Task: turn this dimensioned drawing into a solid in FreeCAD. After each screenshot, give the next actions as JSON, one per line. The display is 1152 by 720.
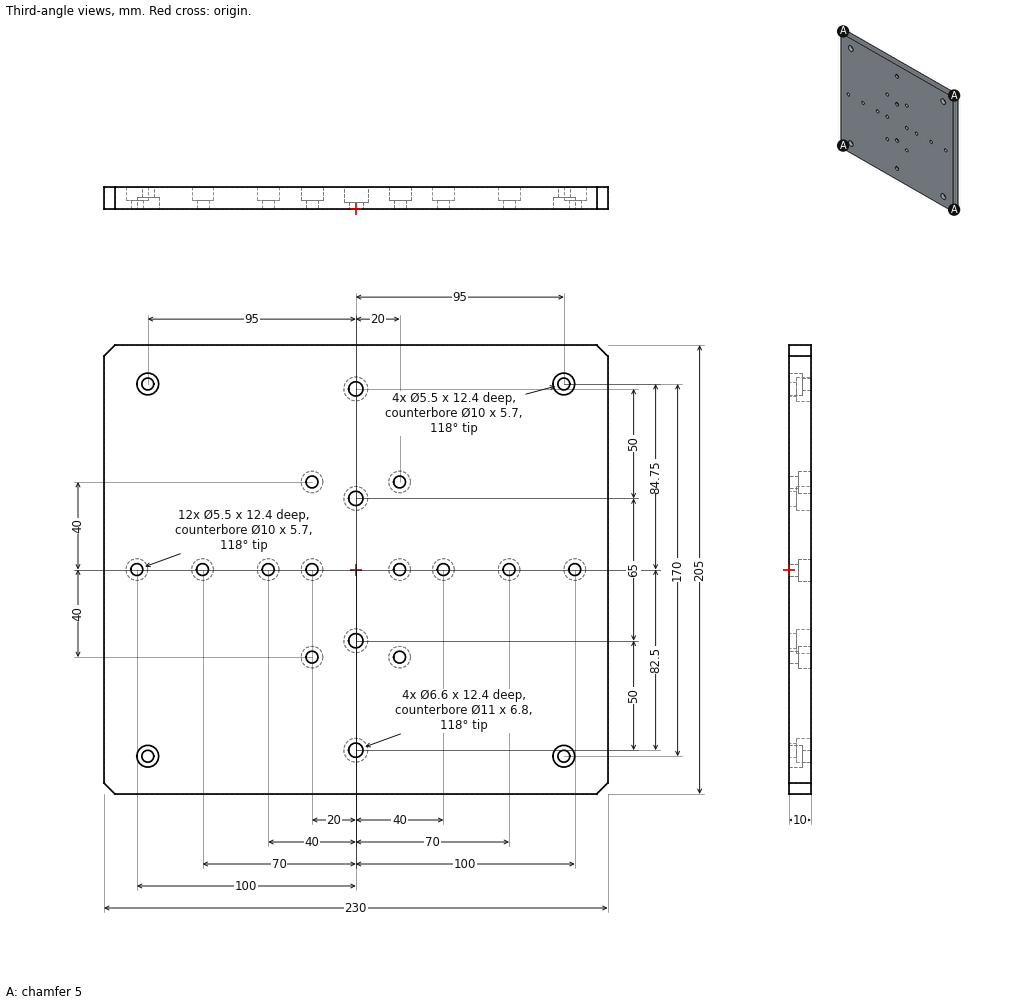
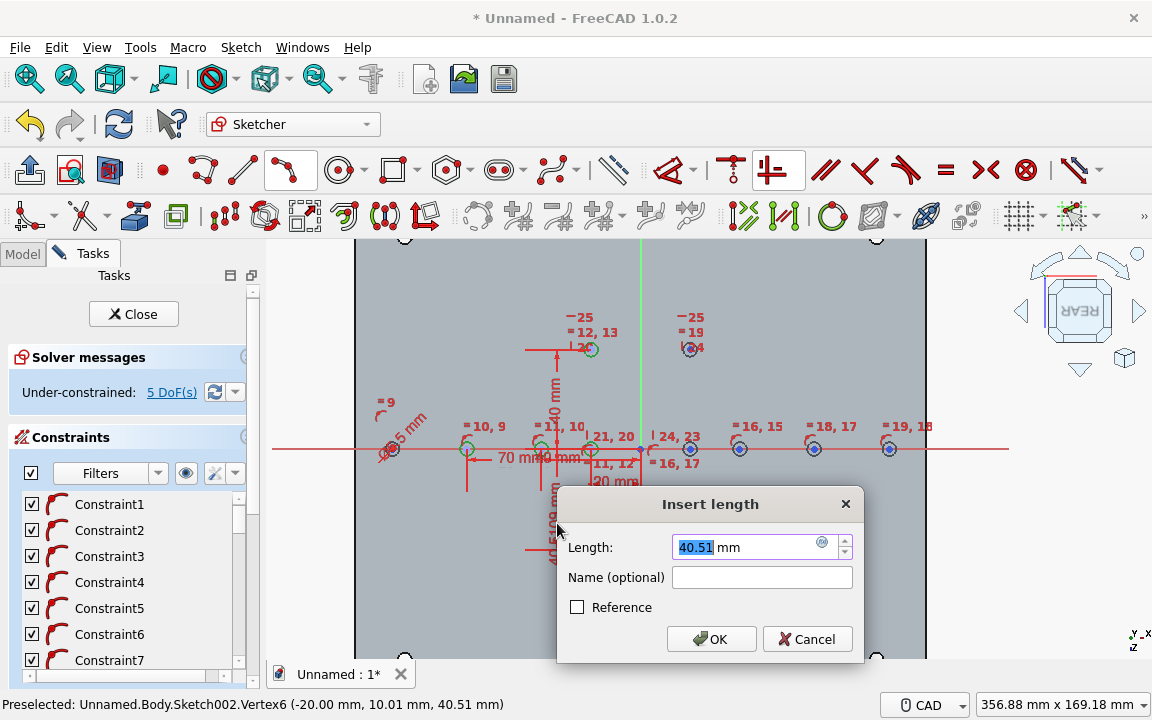
{"action": "type", "text": "40"}
{"action": "key", "text": "Return"}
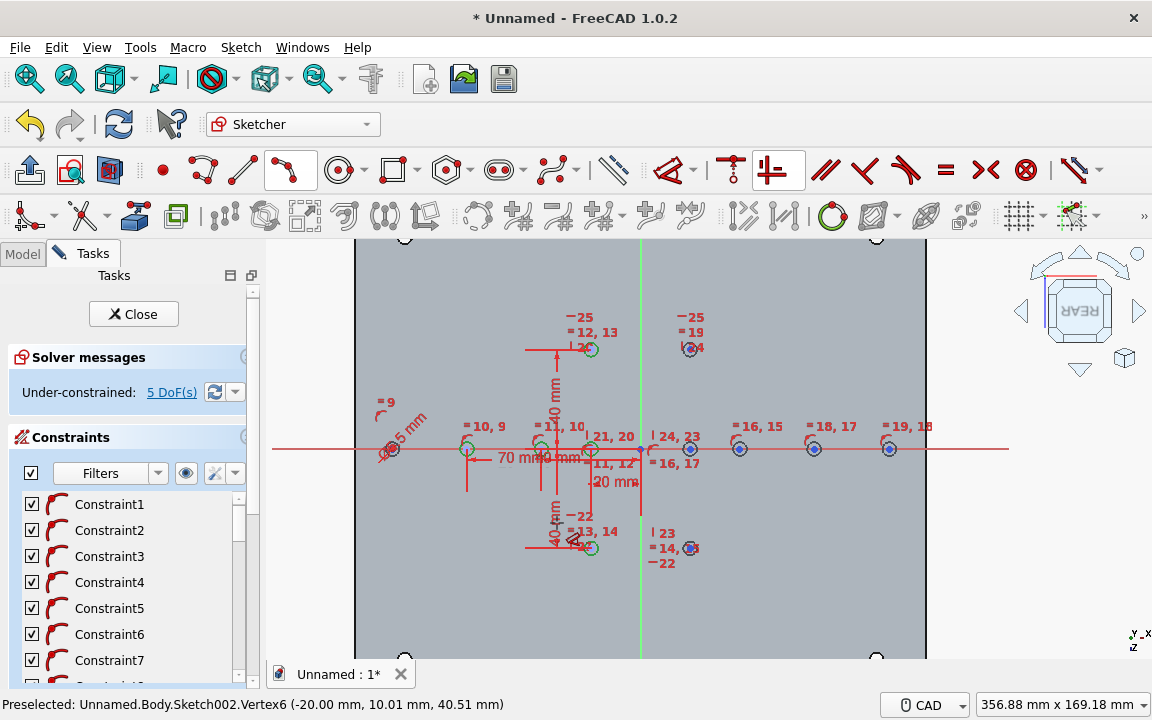
{"action": "left_click", "coordinate": [690, 548]}
{"action": "left_click", "coordinate": [665, 582]}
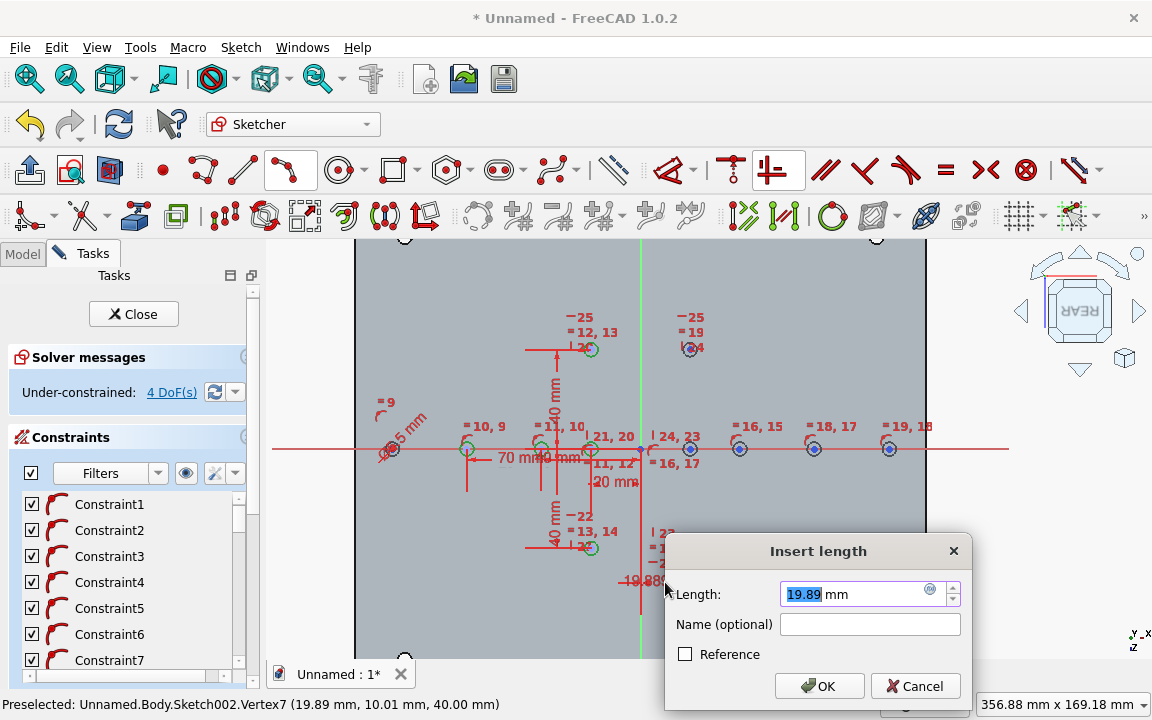
{"action": "type", "text": "20"}
{"action": "key", "text": "Return"}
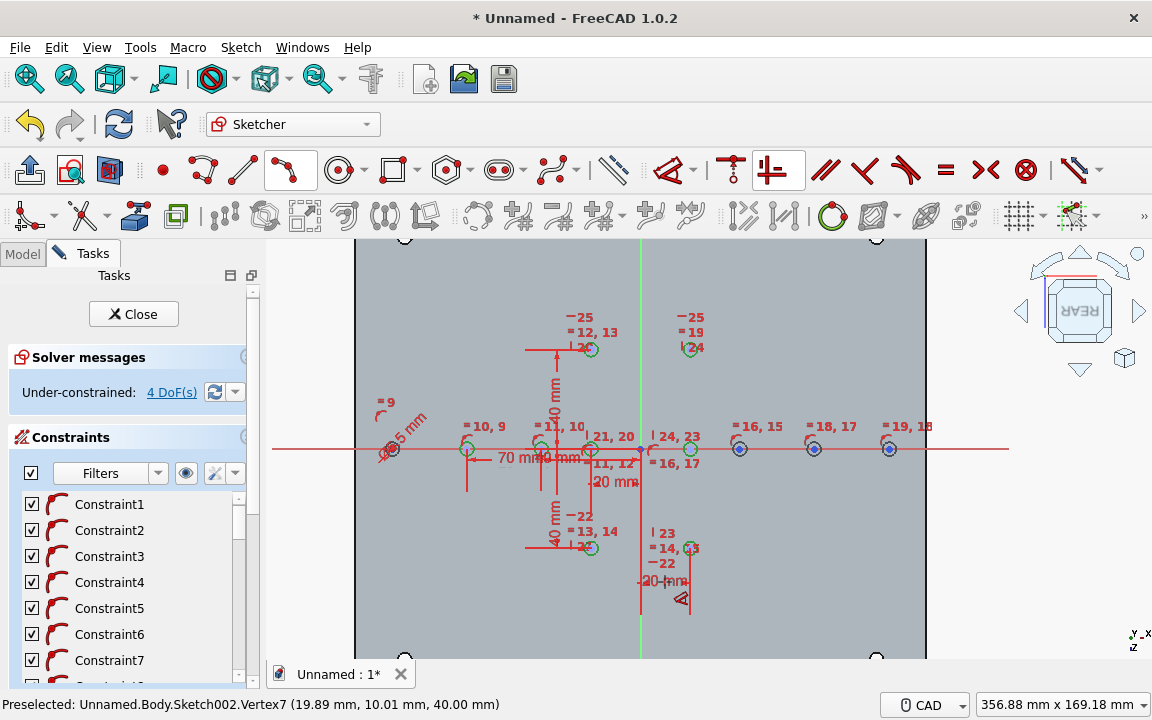
{"action": "left_click", "coordinate": [740, 449]}
{"action": "left_click", "coordinate": [690, 483]}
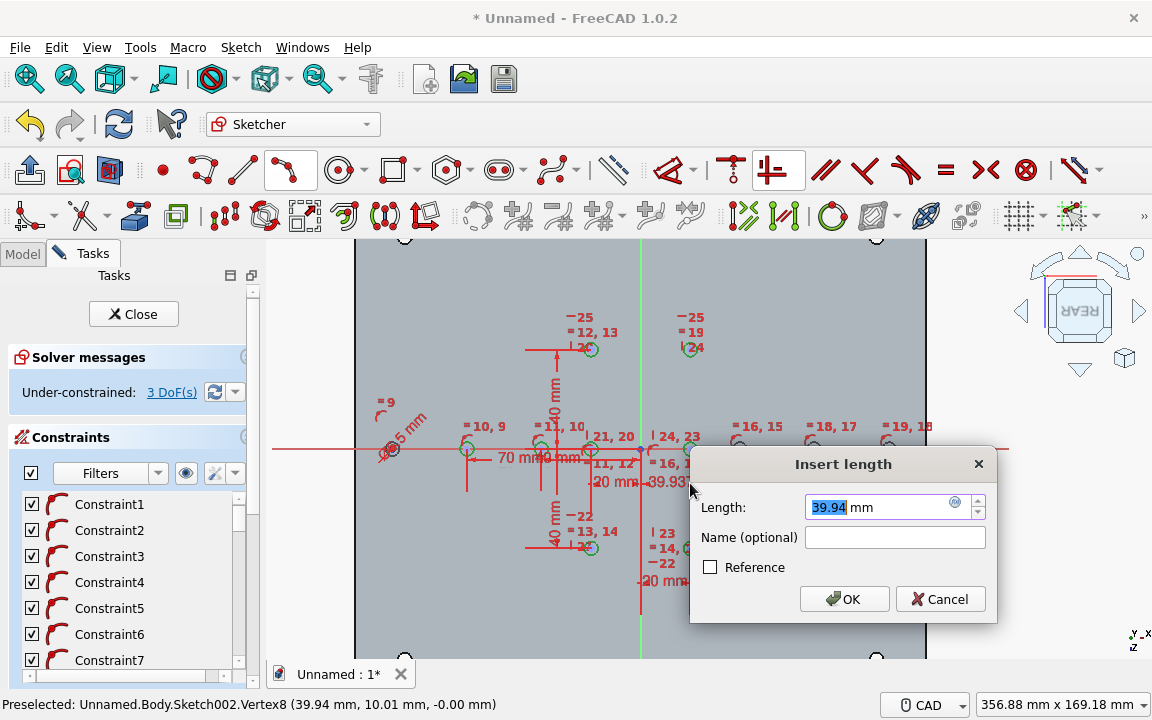
{"action": "type", "text": "40"}
{"action": "key", "text": "Return"}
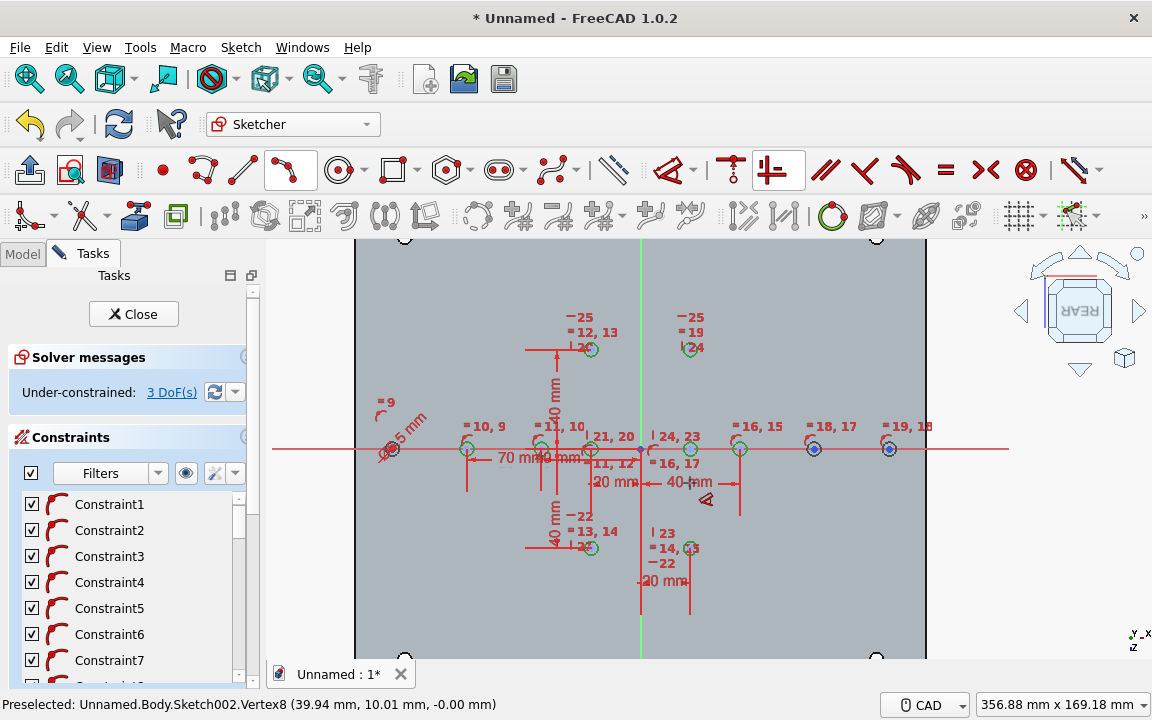
{"action": "left_click", "coordinate": [814, 449]}
{"action": "left_click", "coordinate": [767, 483]}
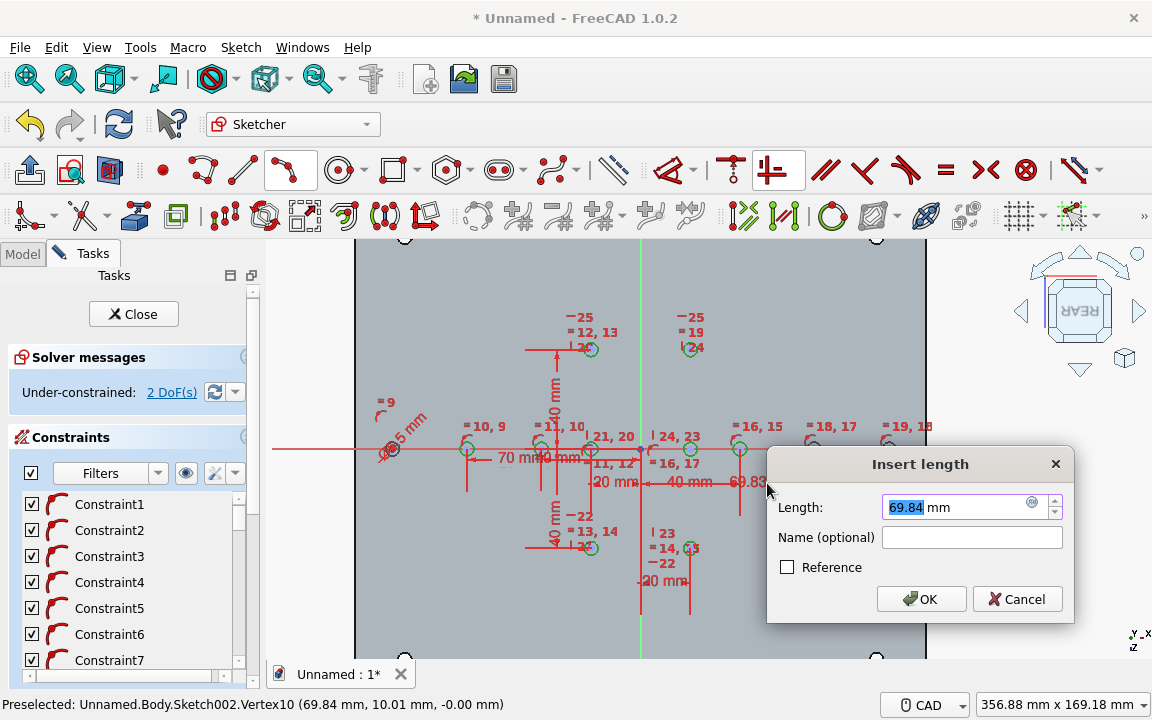
{"action": "type", "text": "70"}
{"action": "key", "text": "Return"}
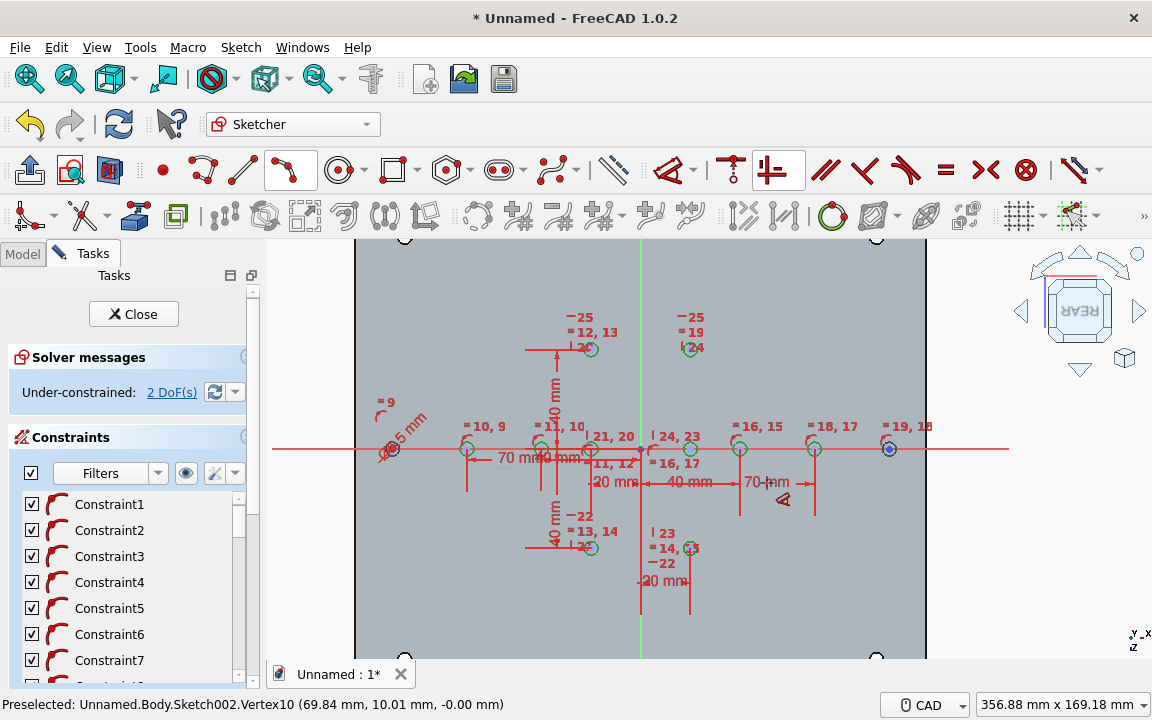
{"action": "left_click", "coordinate": [393, 449]}
{"action": "left_click", "coordinate": [517, 483]}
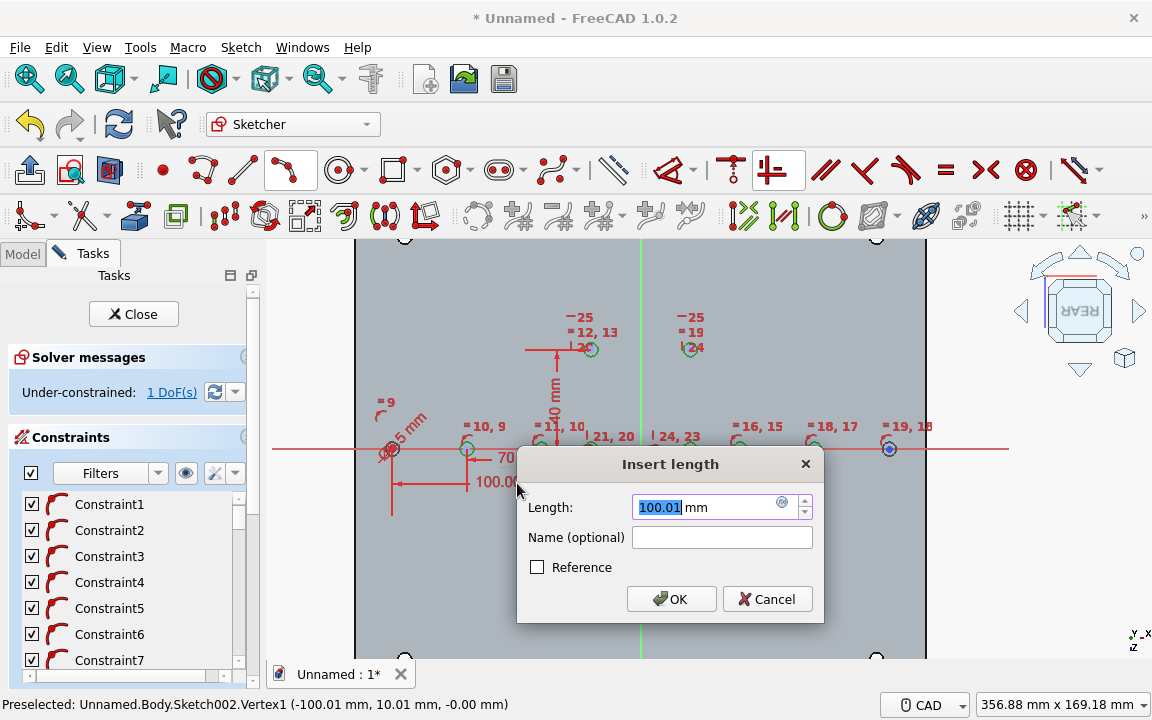
{"action": "type", "text": "100"}
{"action": "key", "text": "Return"}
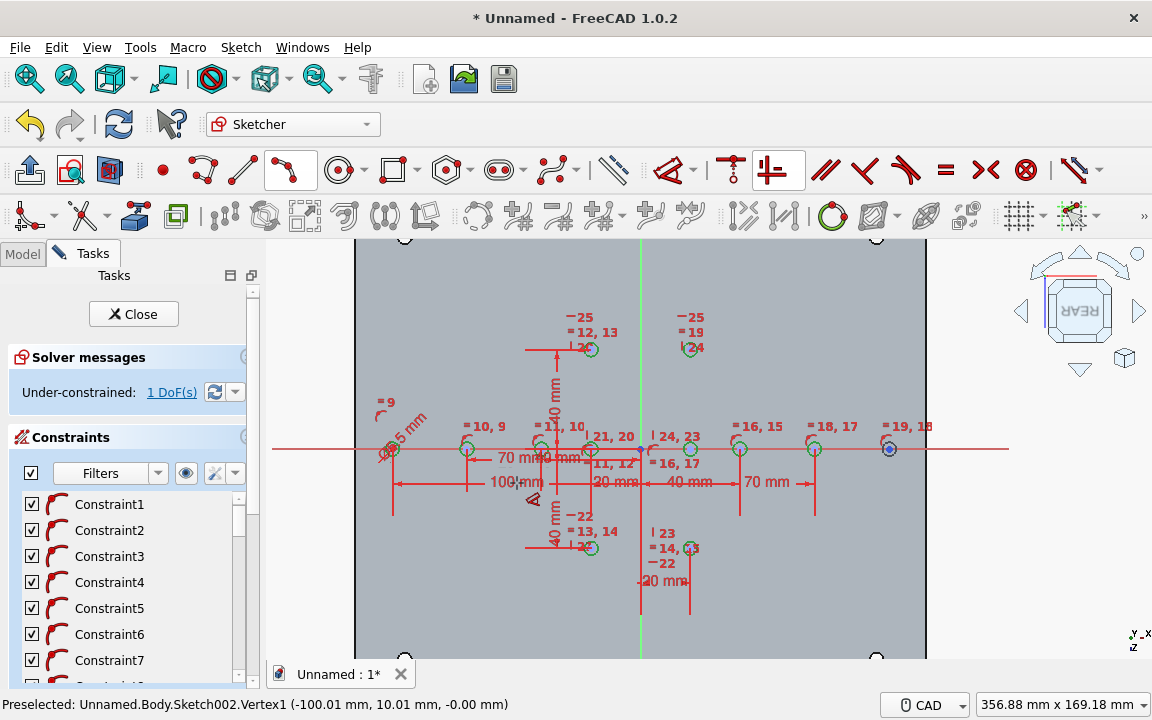
{"action": "left_click", "coordinate": [889, 449]}
{"action": "left_click", "coordinate": [852, 483]}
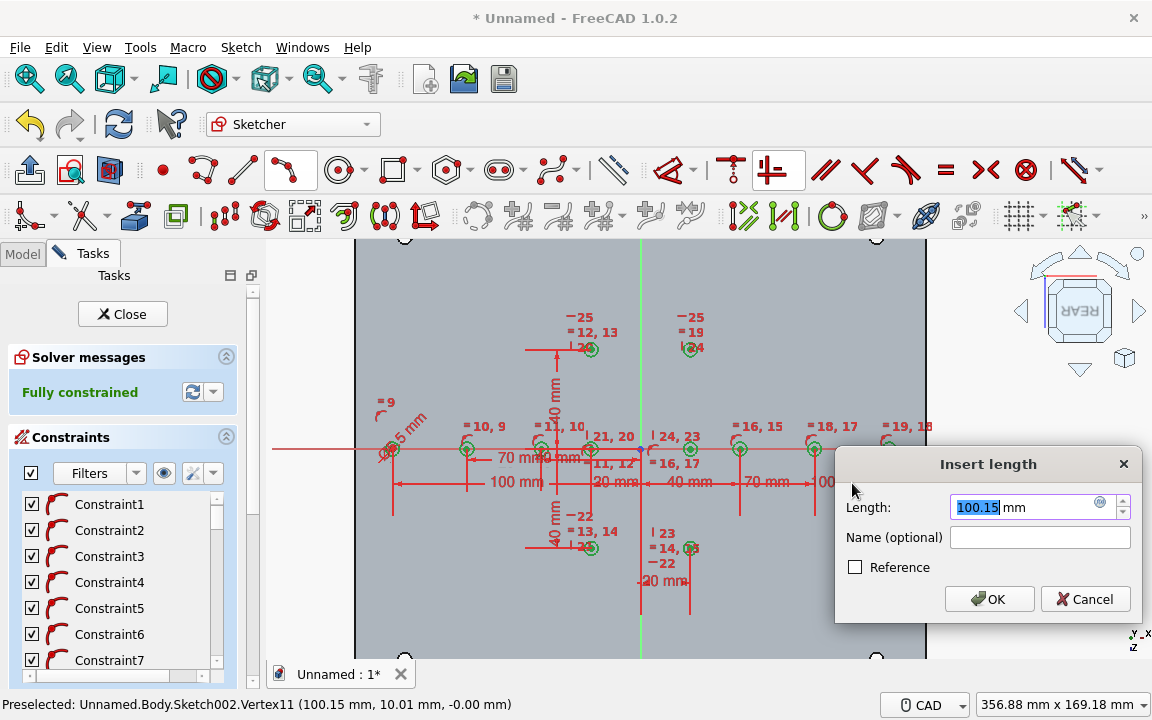
{"action": "type", "text": "100"}
{"action": "key", "text": "Return"}
{"action": "key", "text": "Escape"}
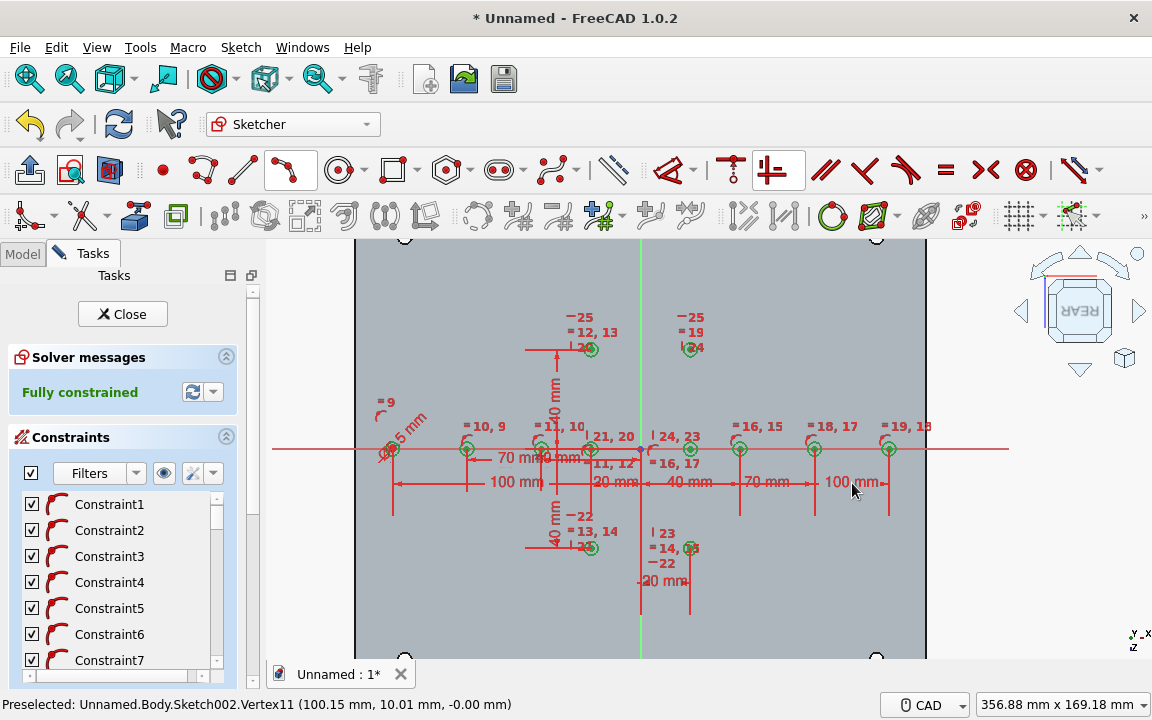
{"action": "left_click", "coordinate": [123, 314]}